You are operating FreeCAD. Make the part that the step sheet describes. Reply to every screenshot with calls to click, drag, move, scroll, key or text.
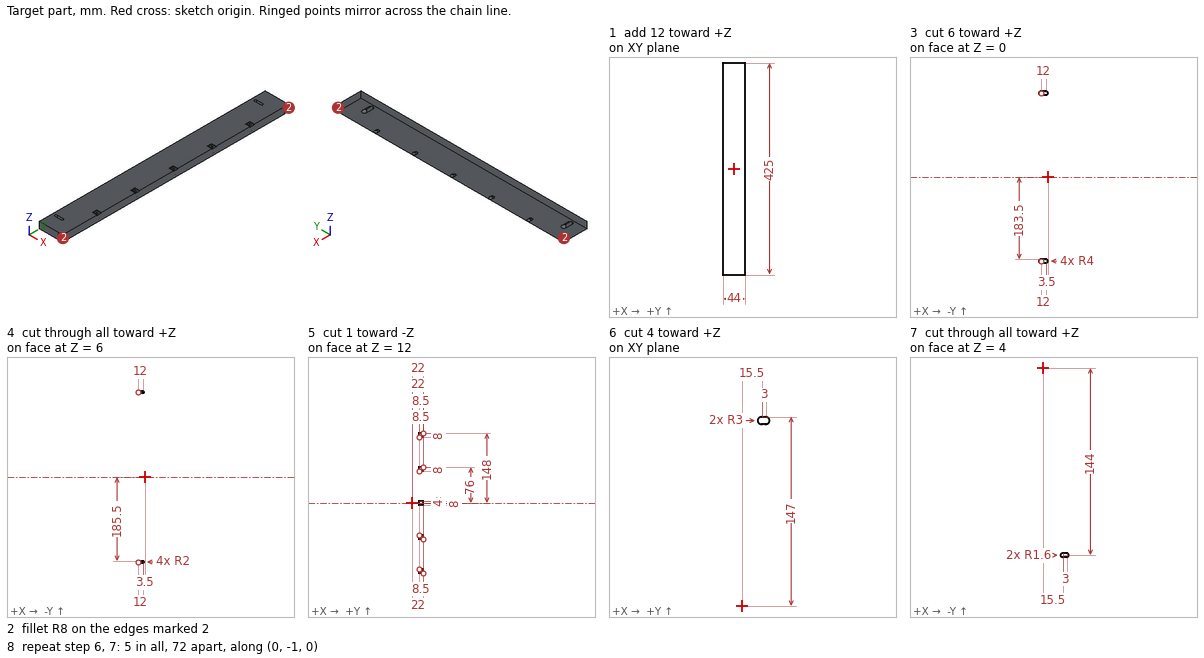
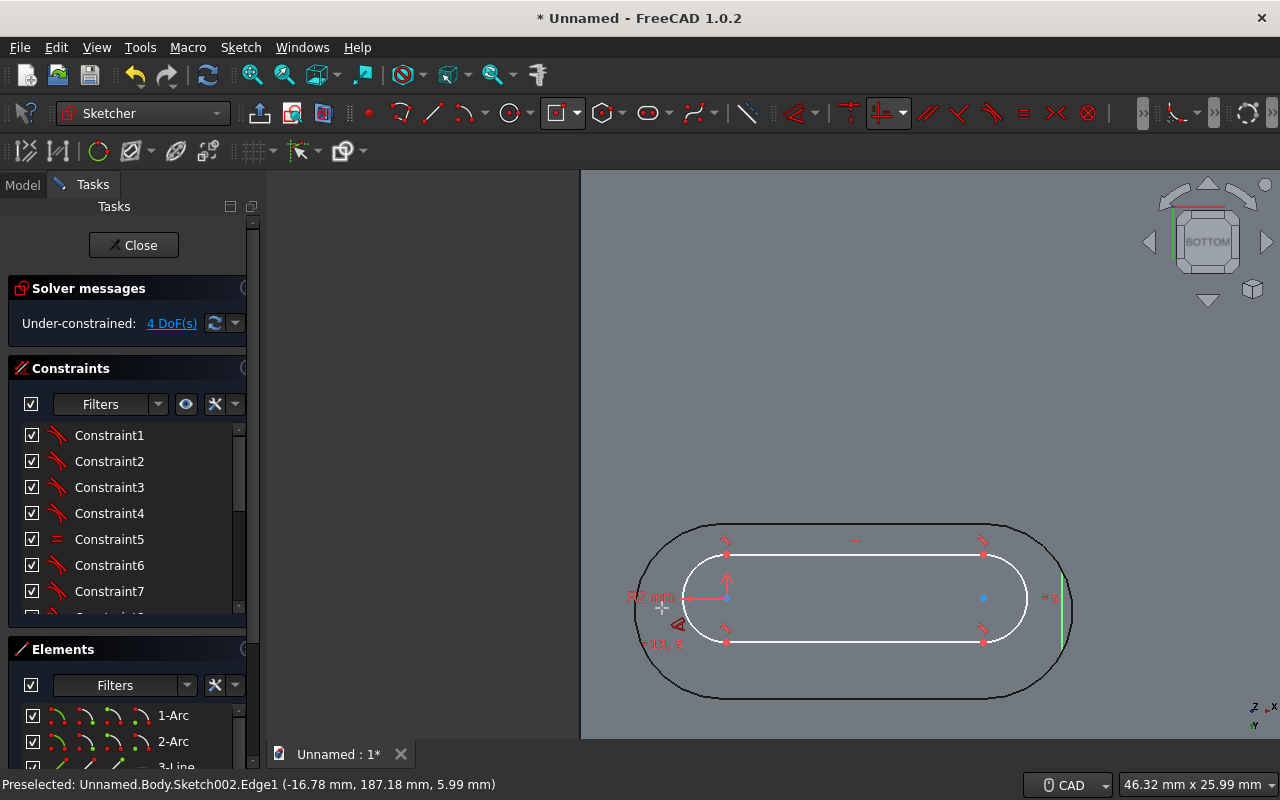
scroll(696, 661, down, 15)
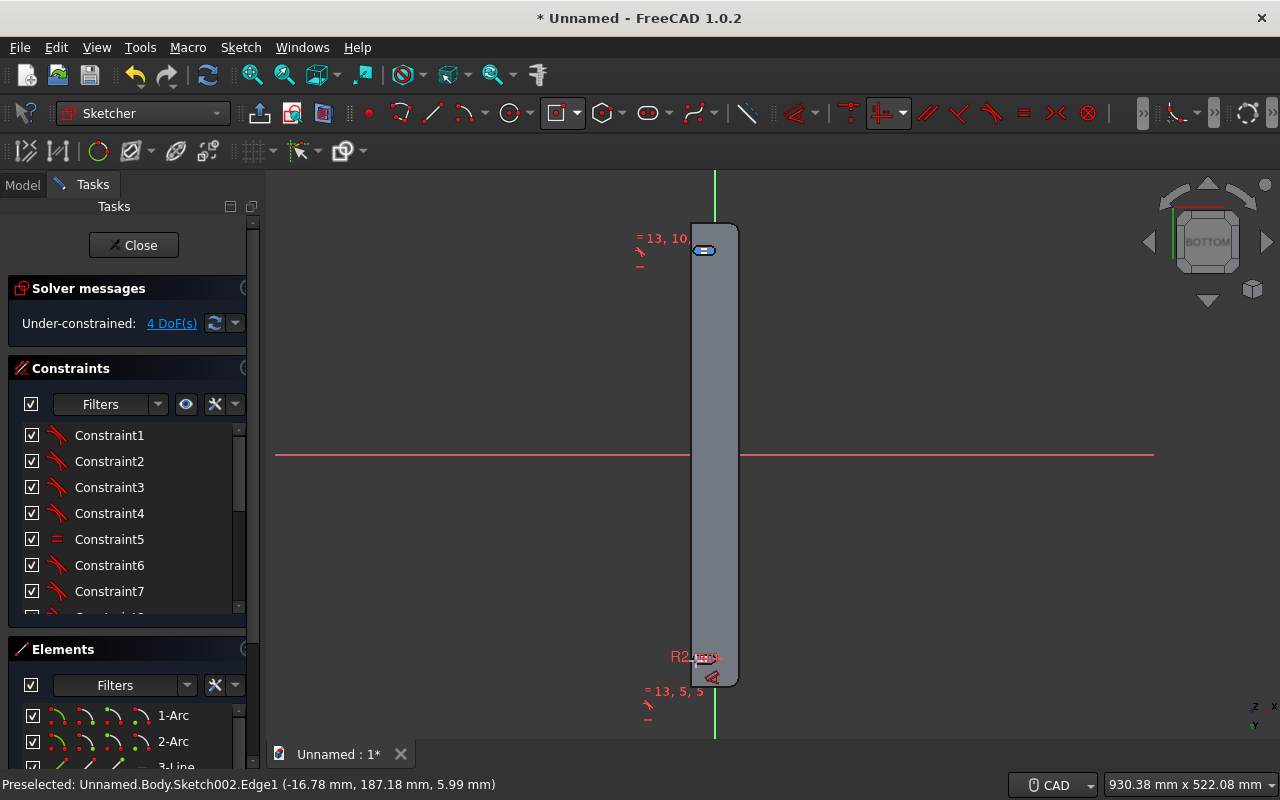
scroll(702, 657, up, 7)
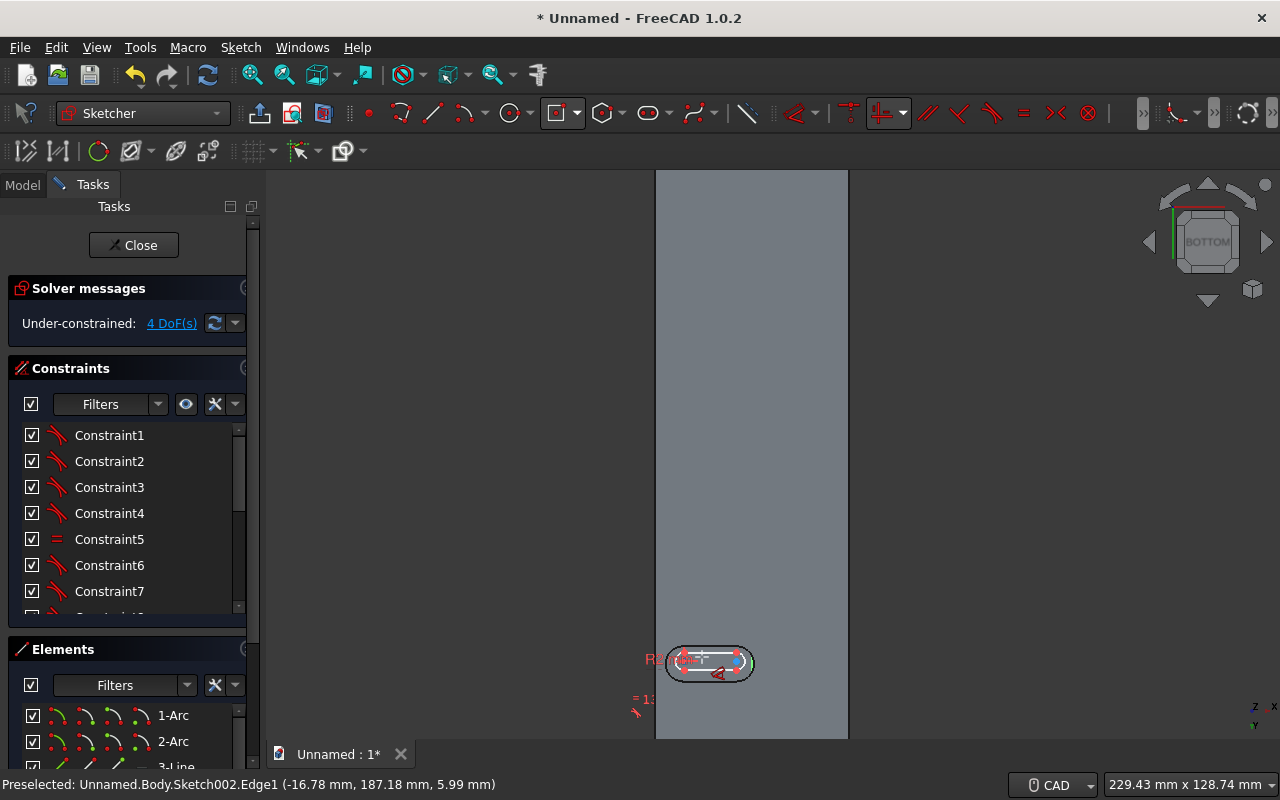
click(700, 653)
click(710, 687)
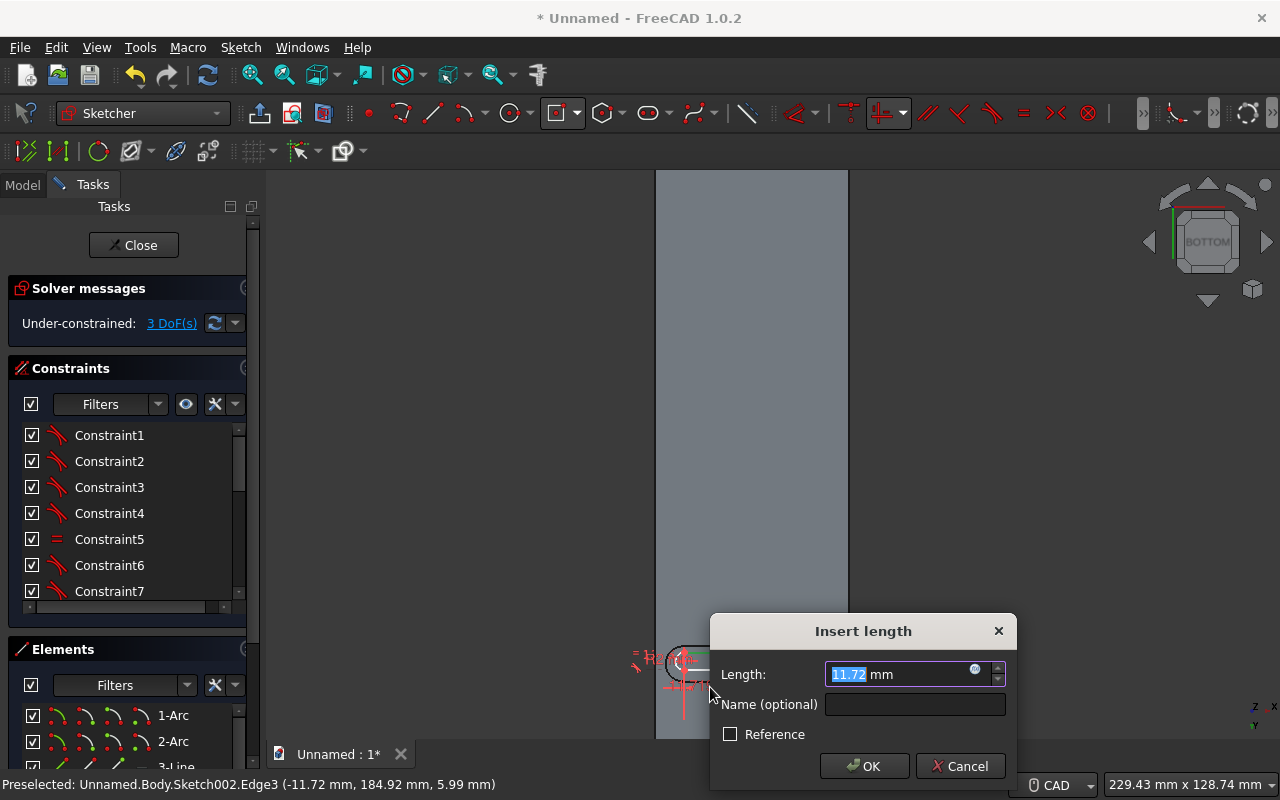
text(12)
key(Return)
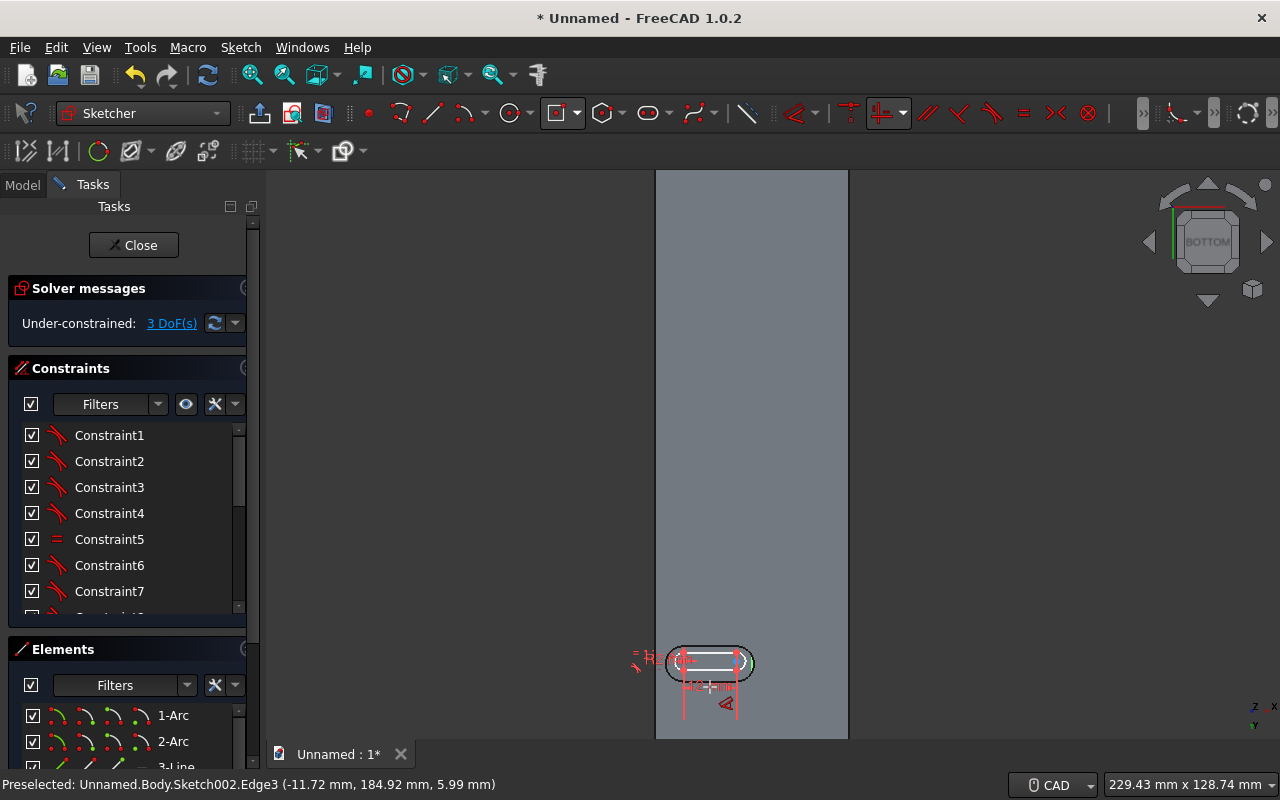
scroll(702, 611, down, 8)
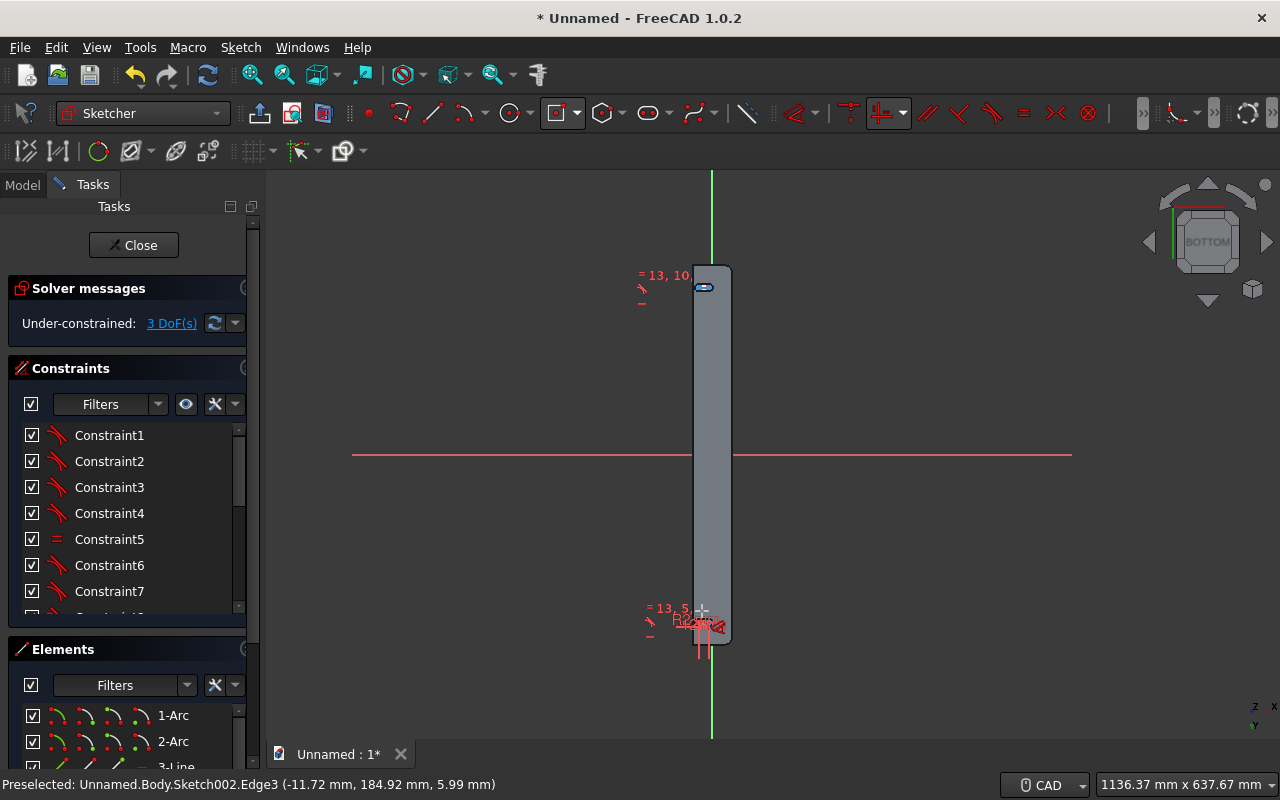
scroll(702, 286, up, 8)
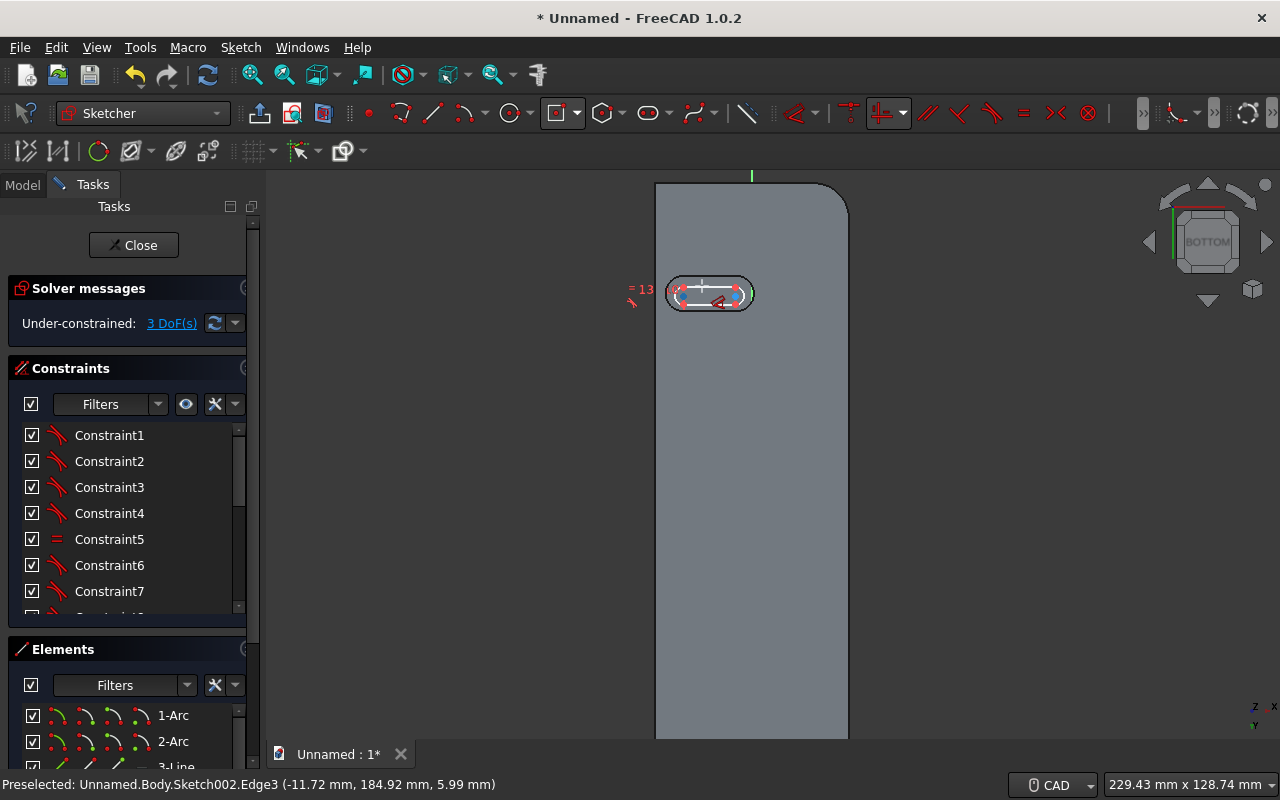
click(699, 287)
click(709, 253)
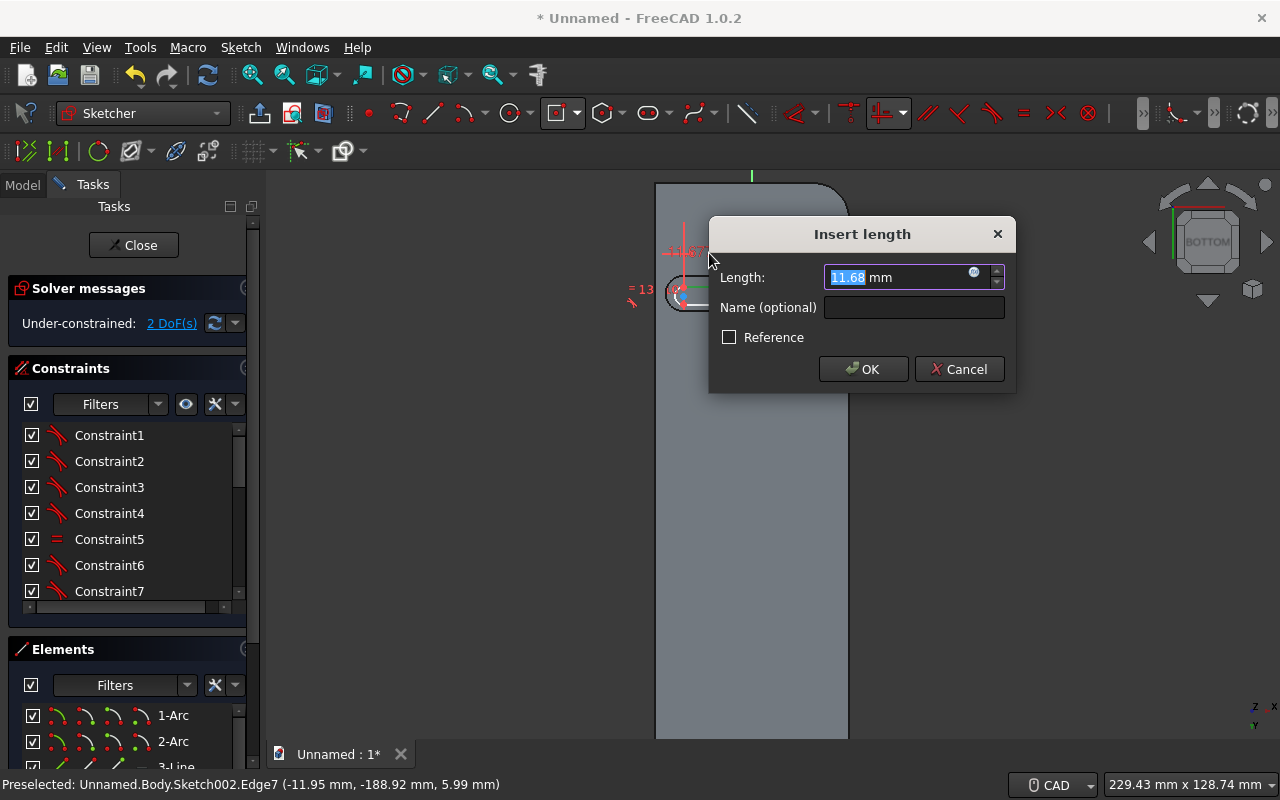
text(12)
key(Return)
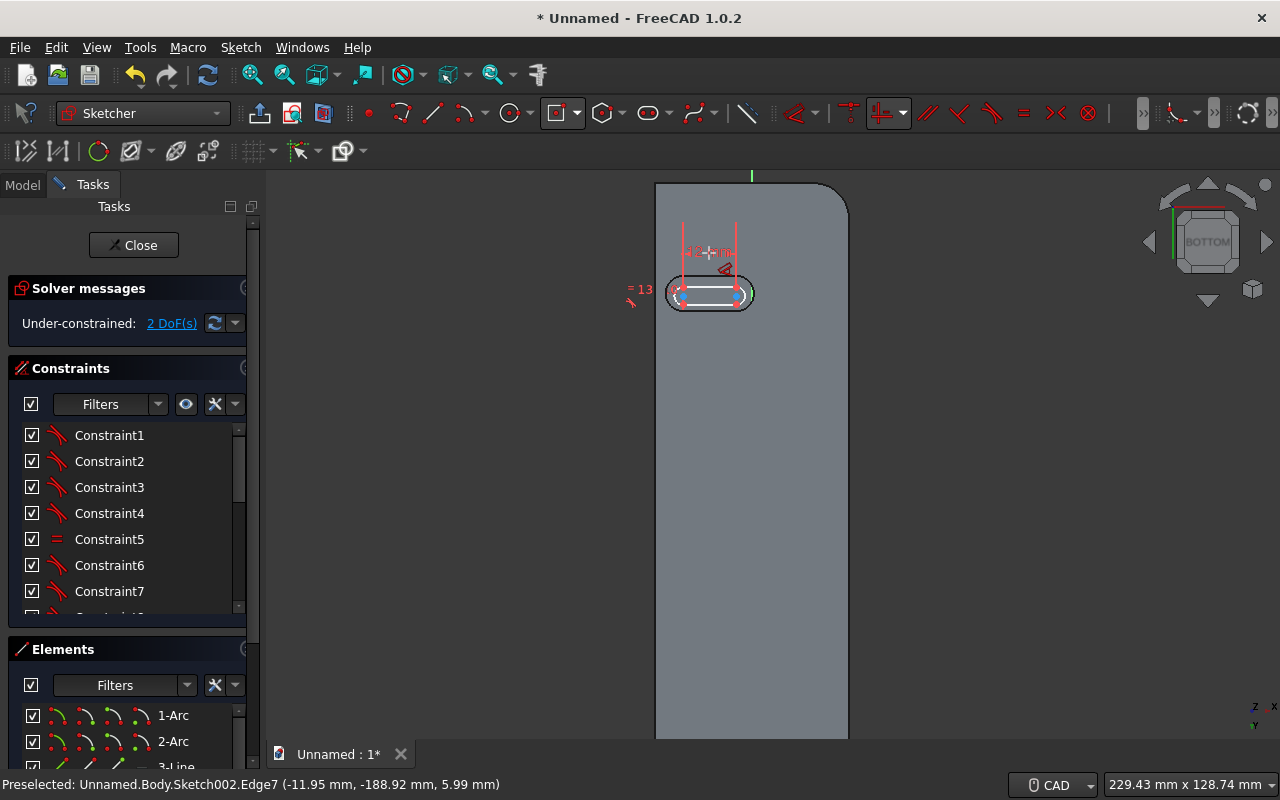
scroll(702, 286, down, 8)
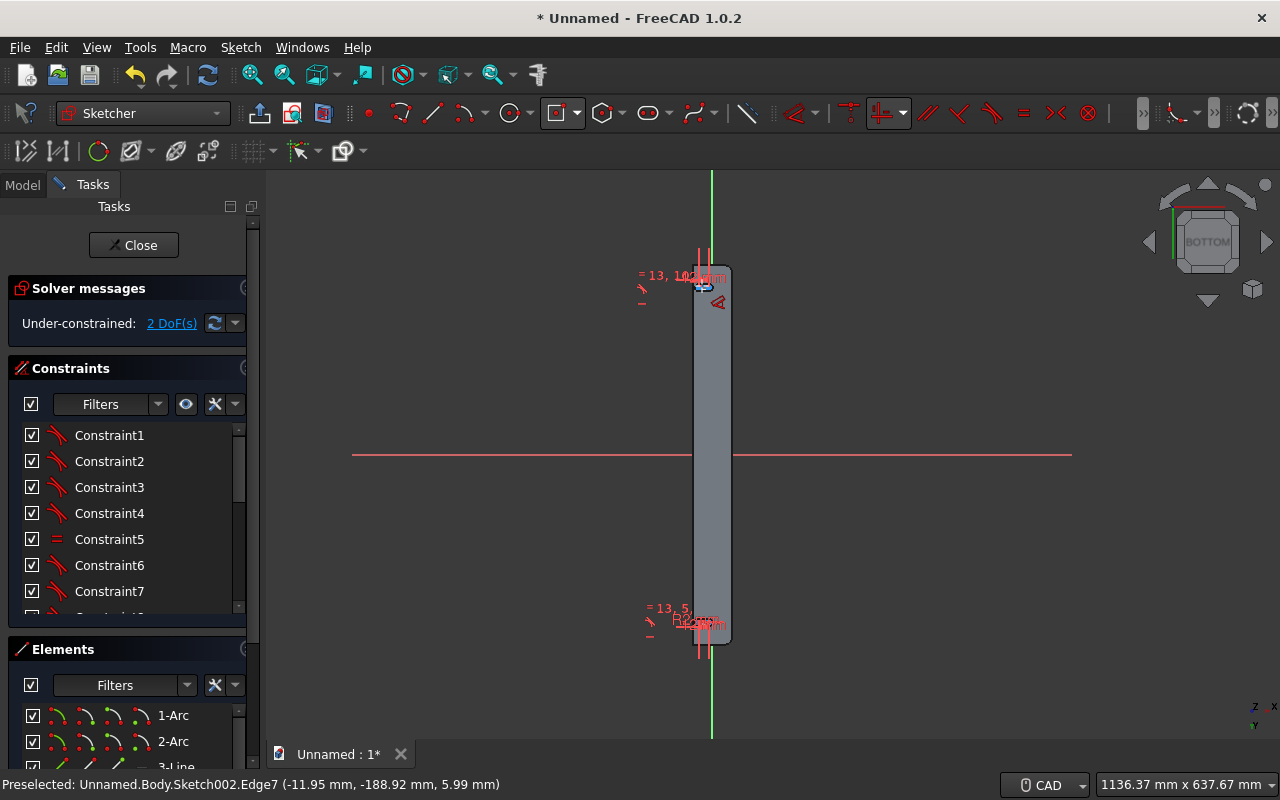
scroll(709, 624, up, 13)